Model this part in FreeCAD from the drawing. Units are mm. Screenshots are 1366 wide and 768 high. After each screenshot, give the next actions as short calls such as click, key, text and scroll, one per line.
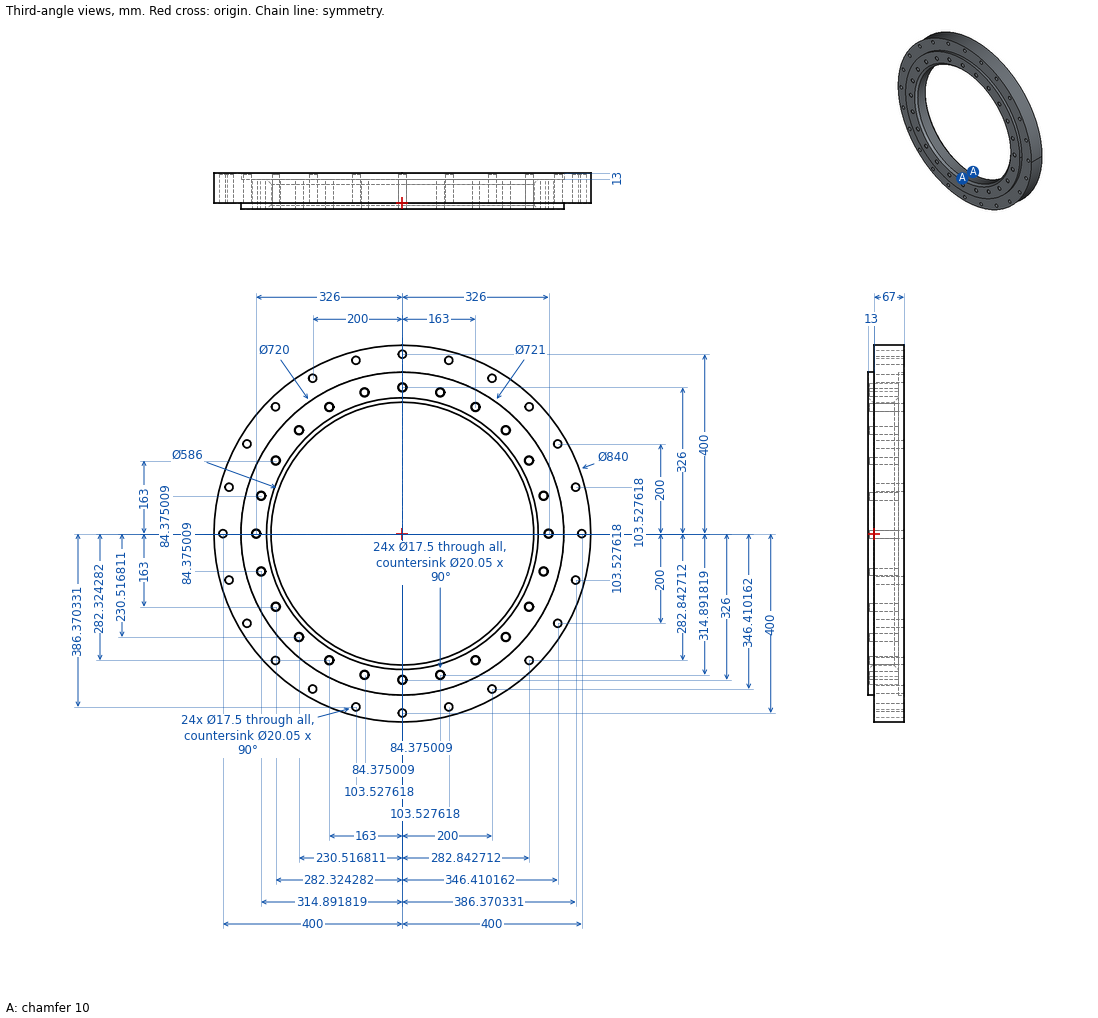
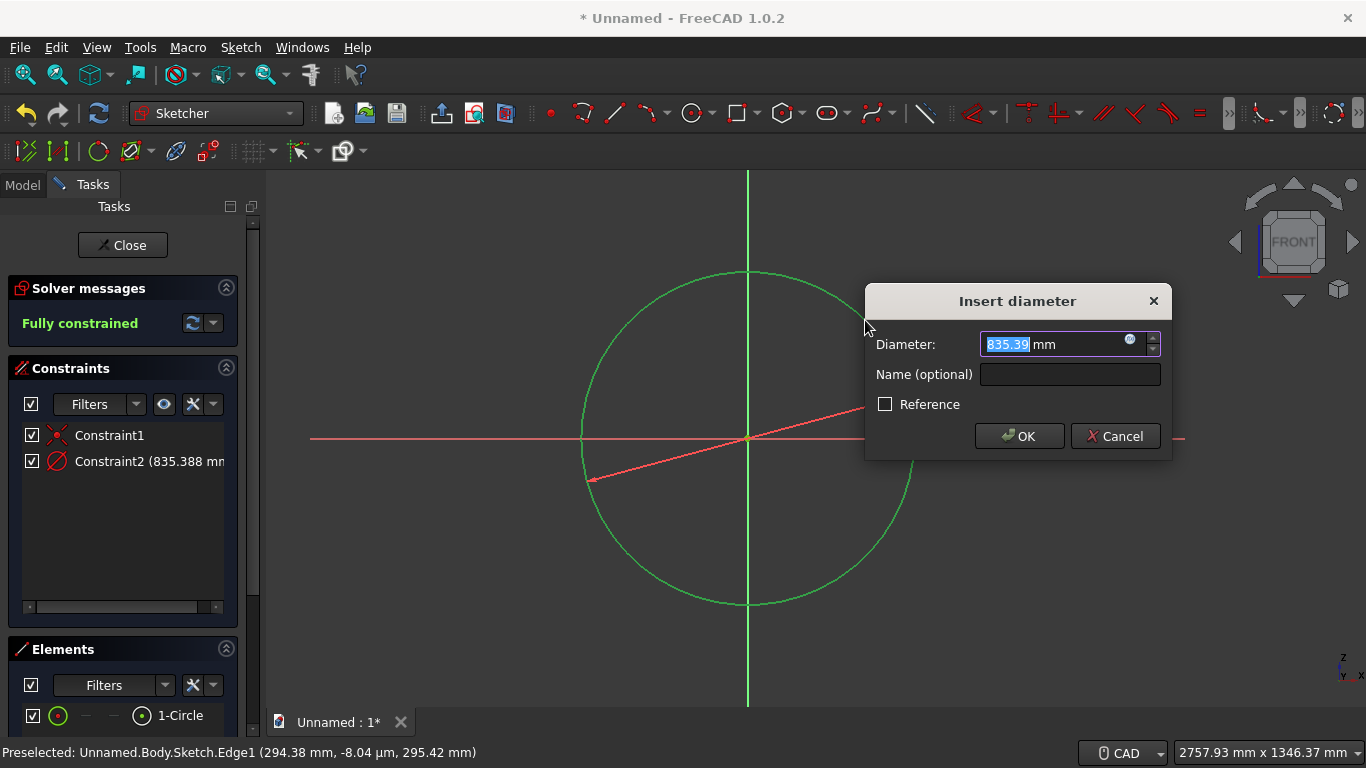
text(840)
key(Return)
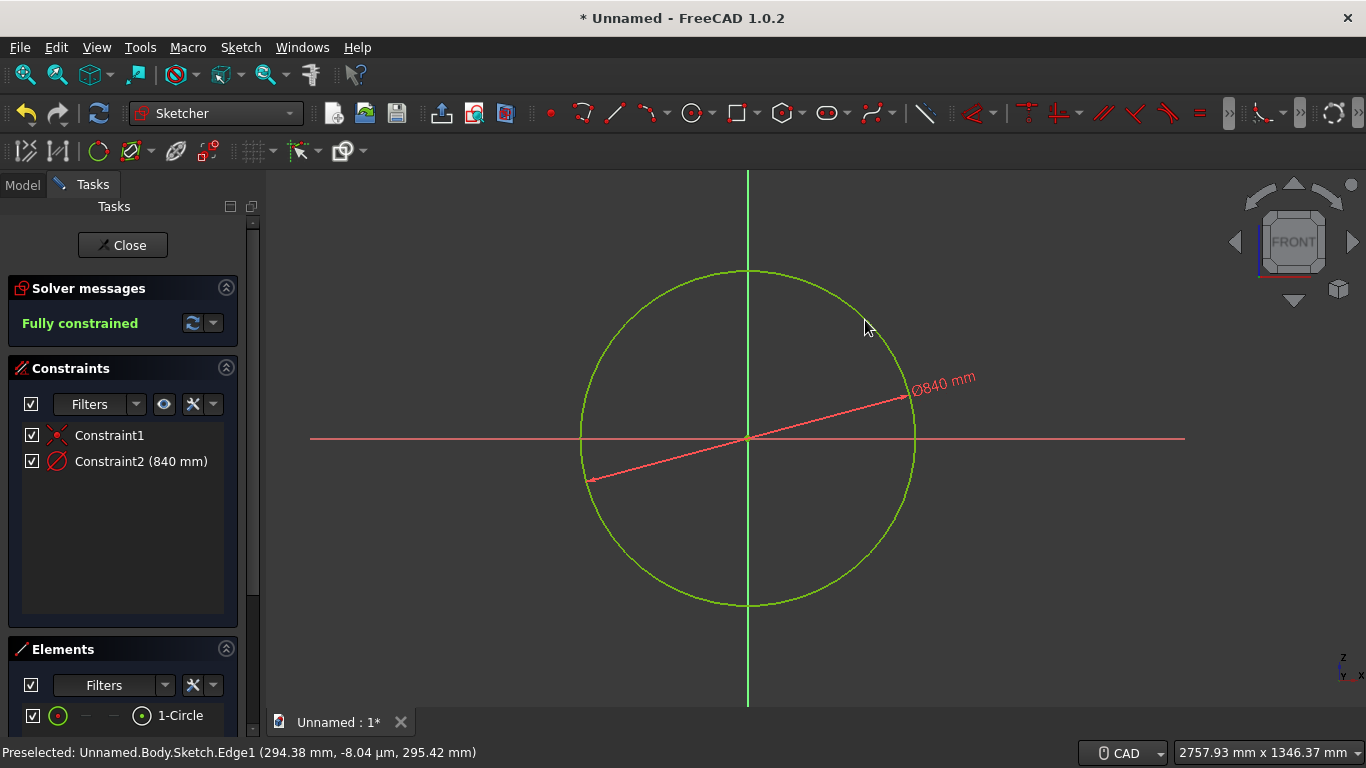
click(123, 245)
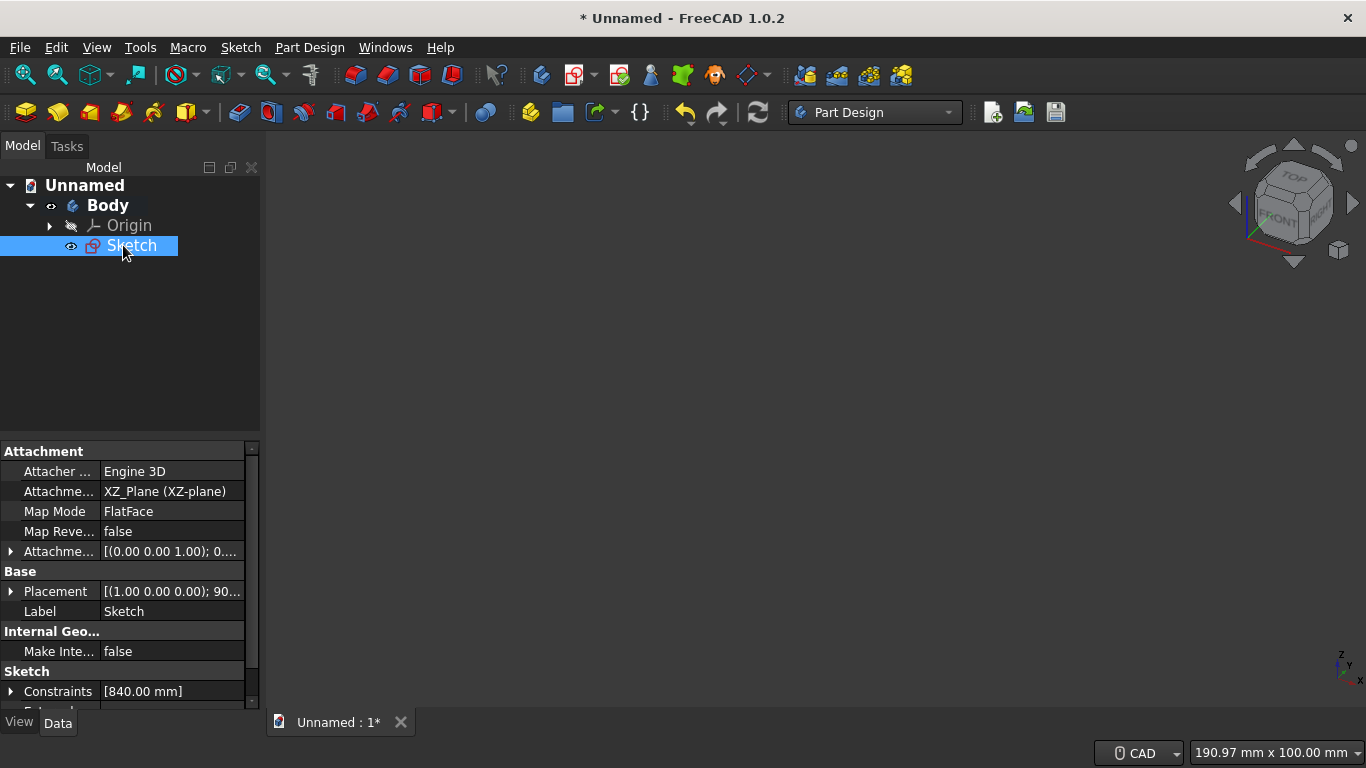
click(26, 112)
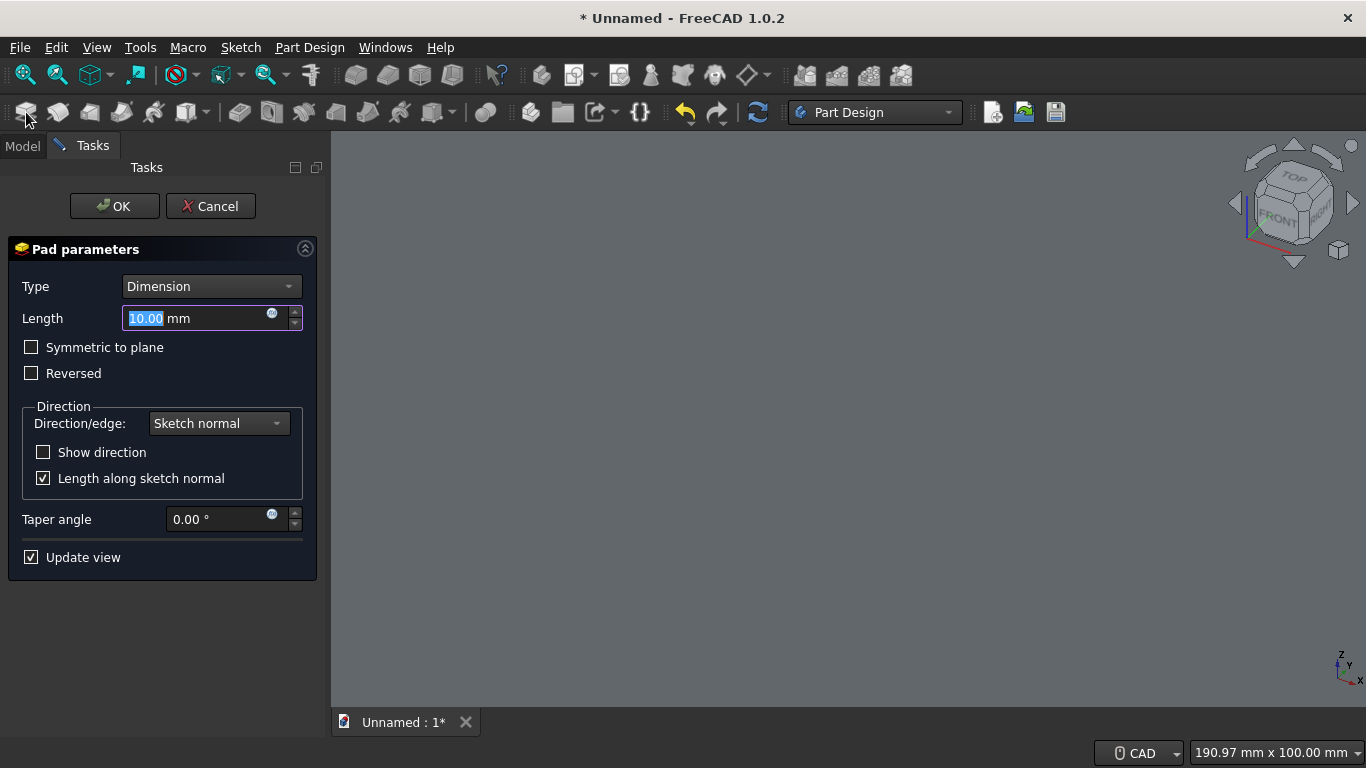
text(67)
key(Tab)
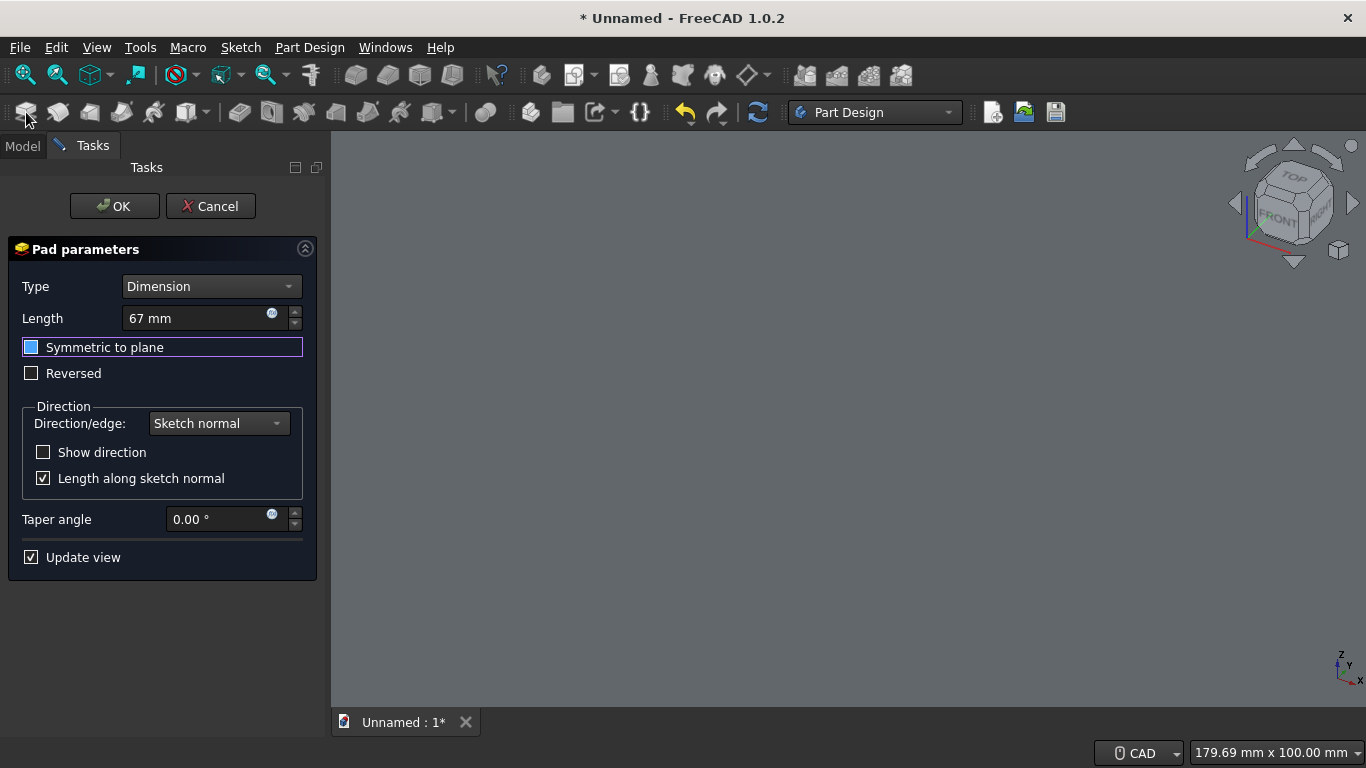
click(30, 373)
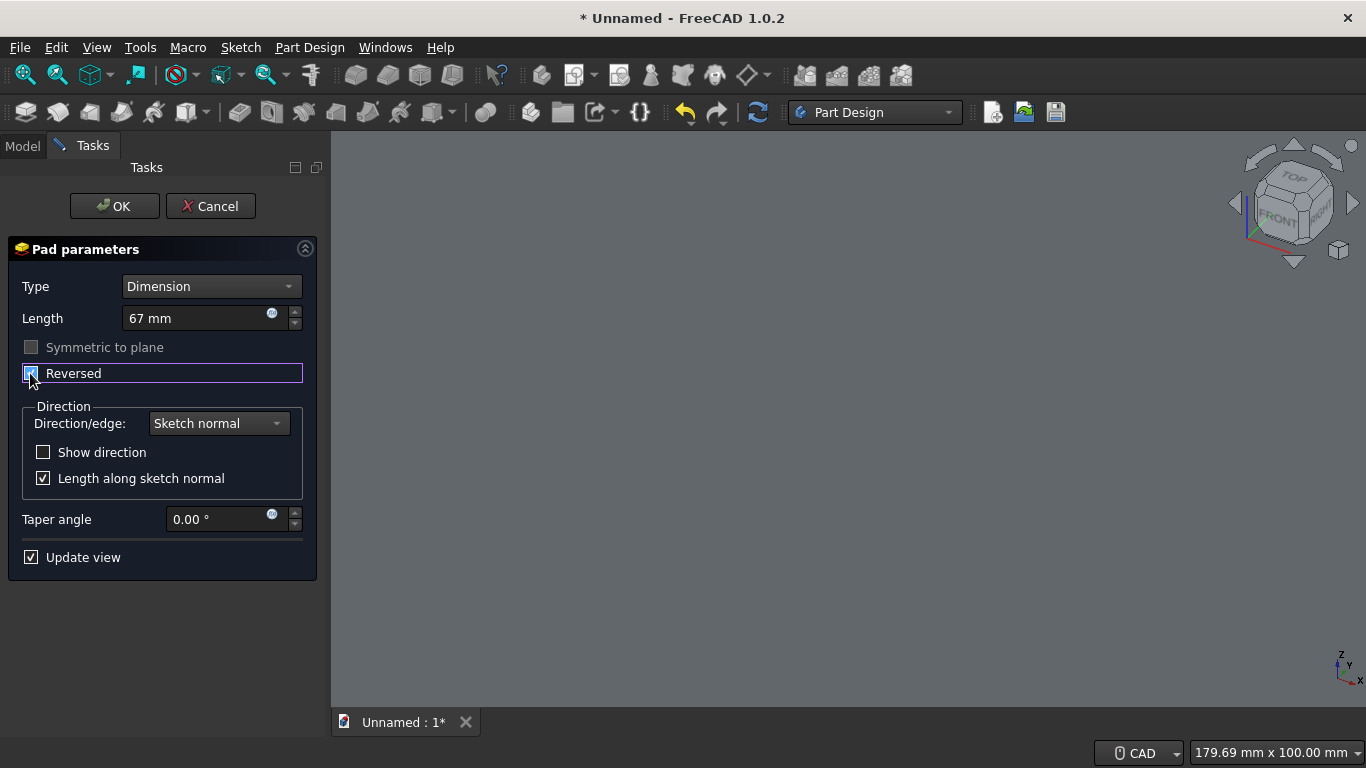
click(115, 206)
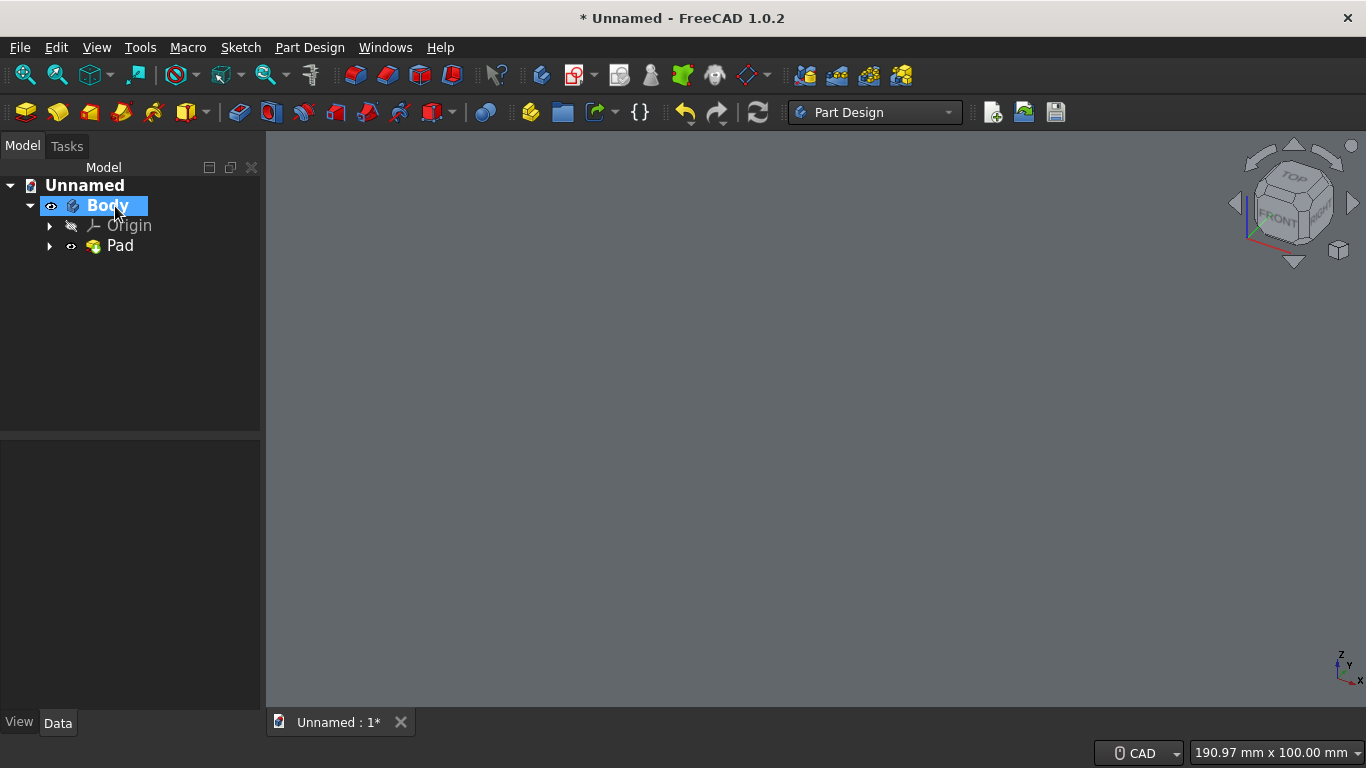
click(26, 76)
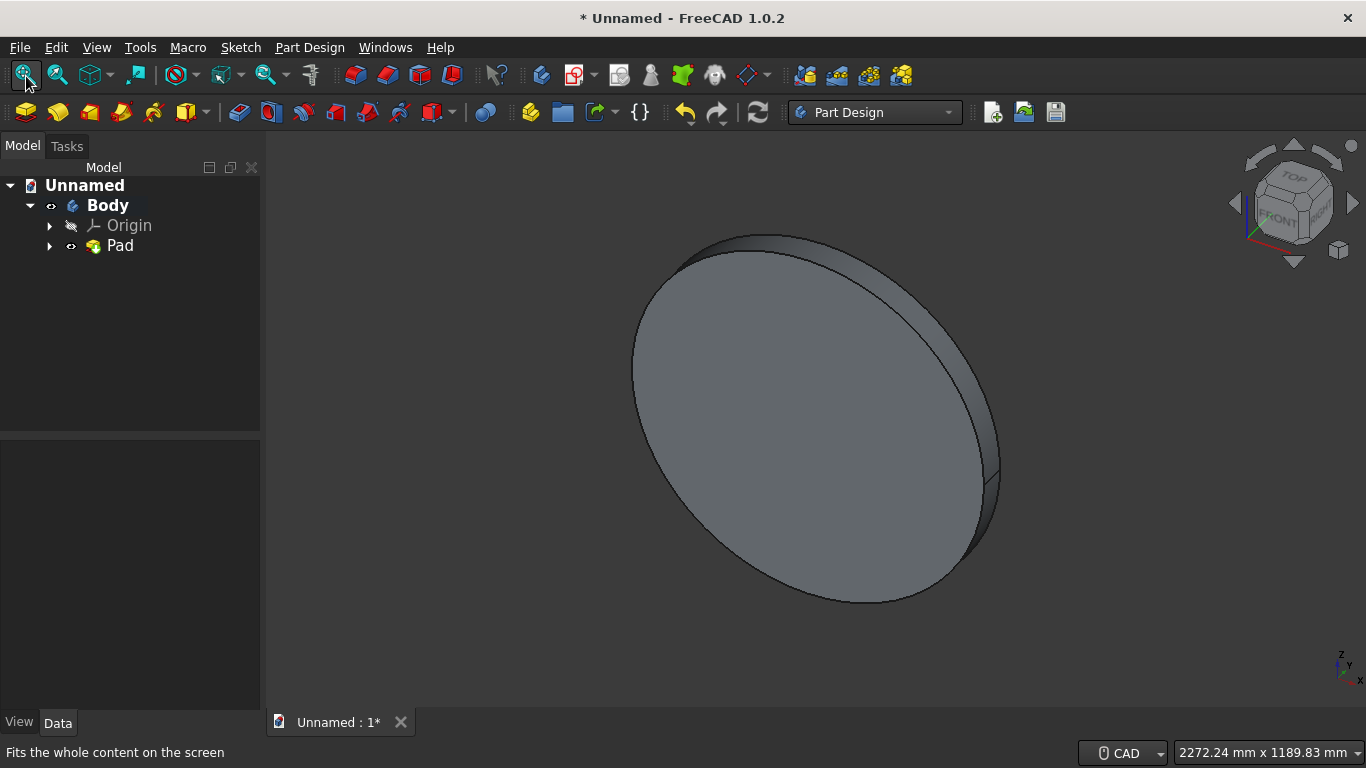
key(4)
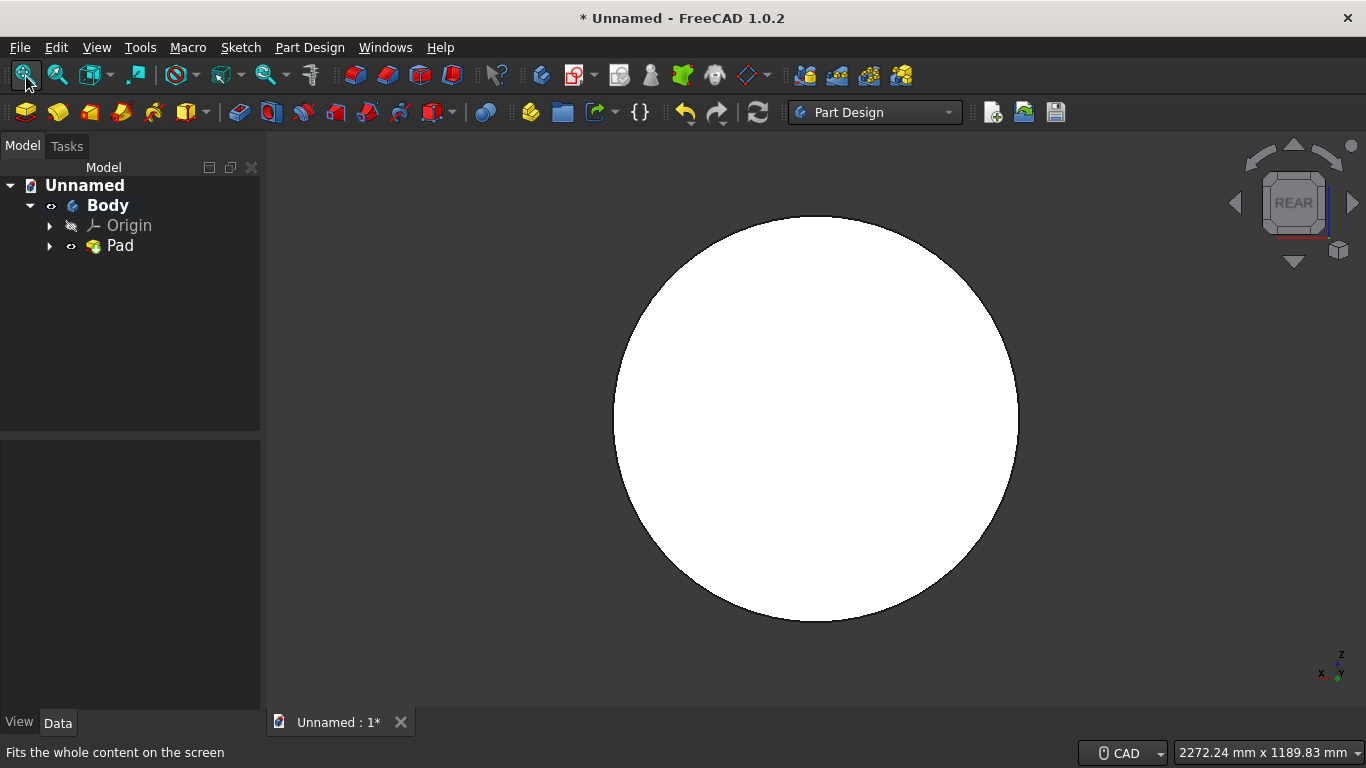
click(816, 418)